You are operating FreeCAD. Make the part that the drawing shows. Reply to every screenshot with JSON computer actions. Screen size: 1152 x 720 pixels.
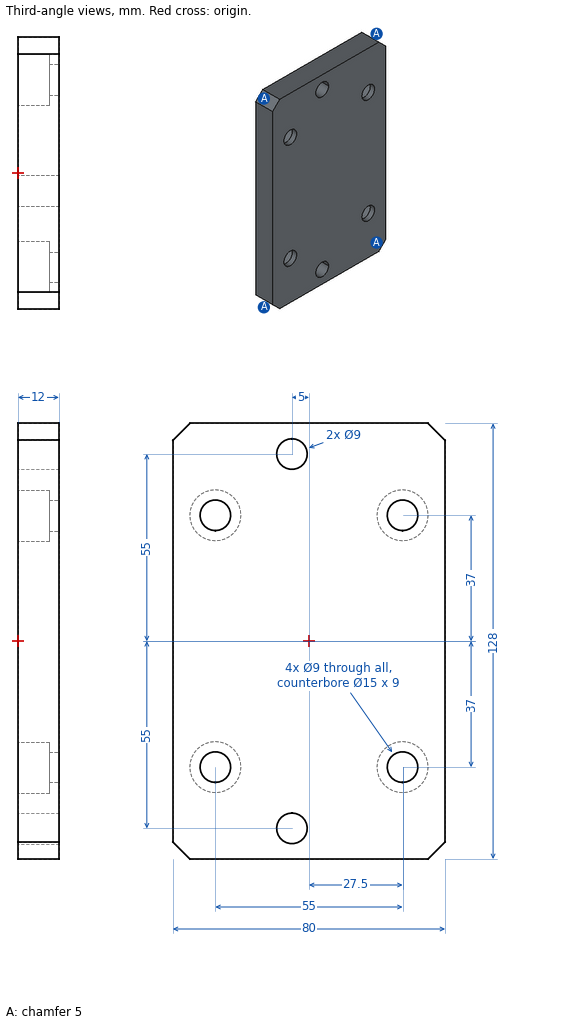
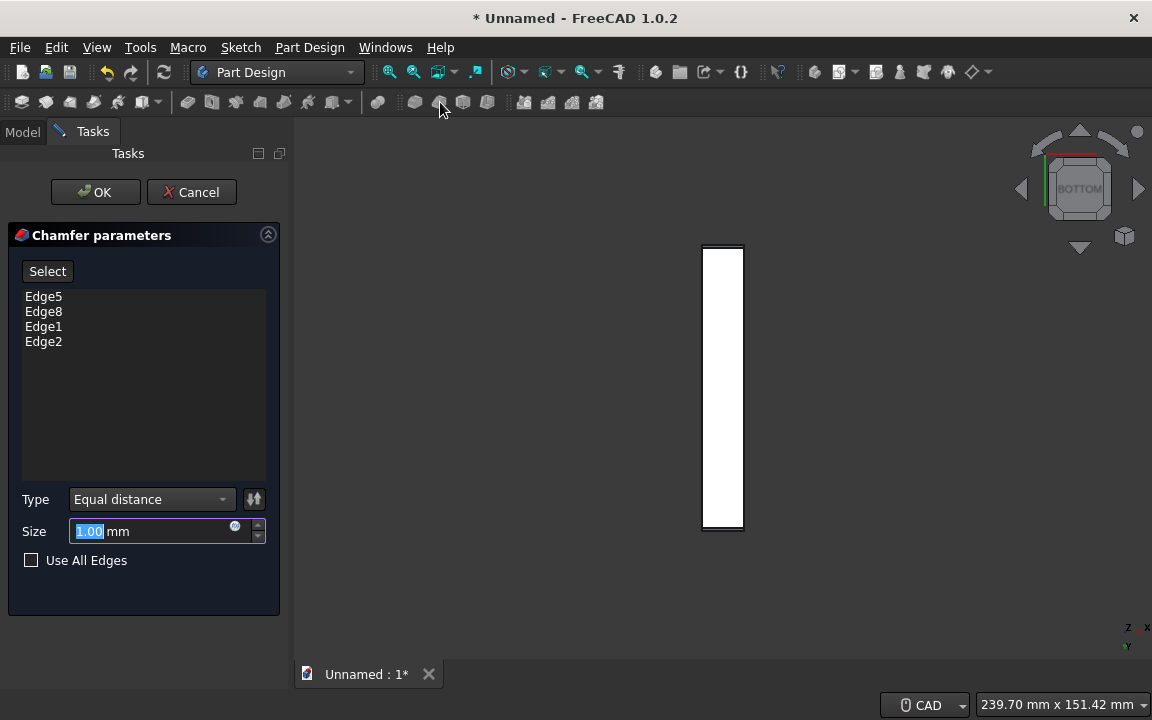
{"action": "type", "text": "5"}
{"action": "key", "text": "Tab"}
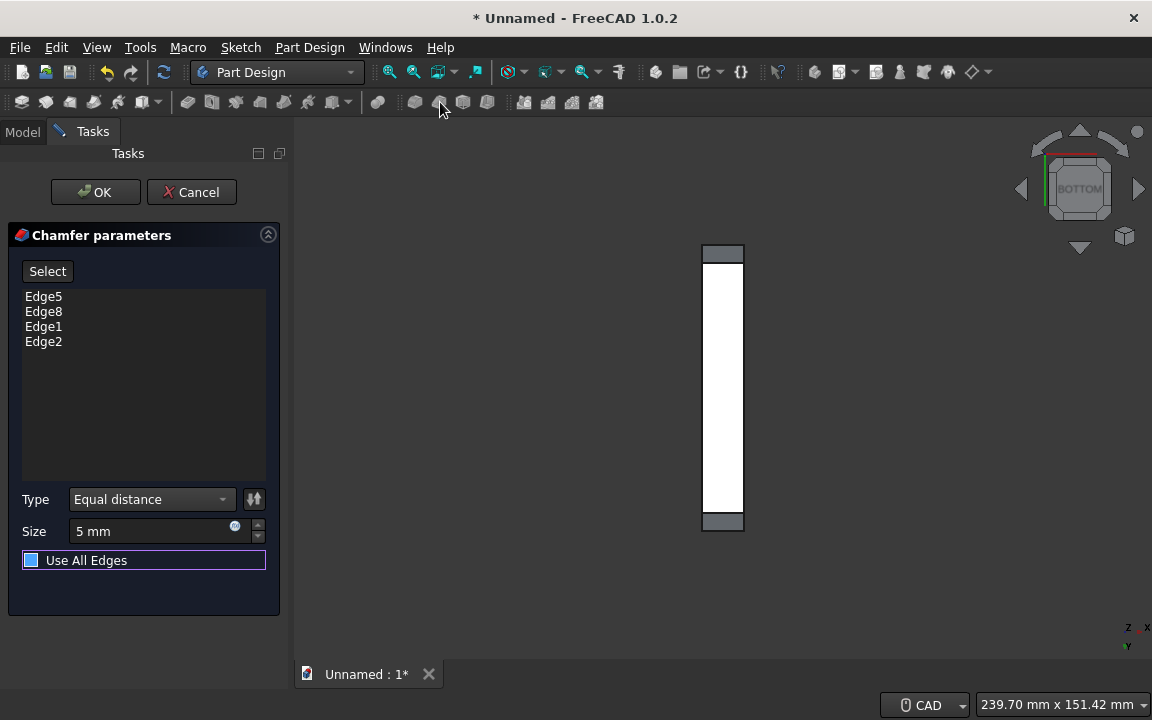
{"action": "left_click", "coordinate": [96, 192]}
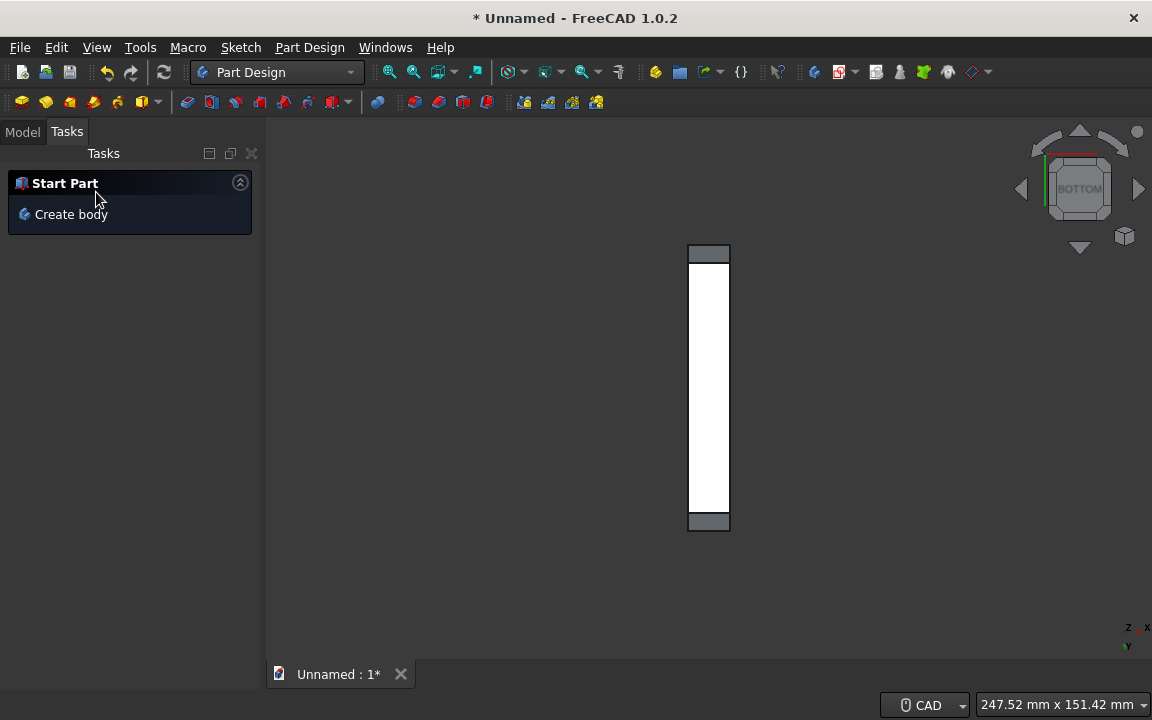
{"action": "key", "text": "0"}